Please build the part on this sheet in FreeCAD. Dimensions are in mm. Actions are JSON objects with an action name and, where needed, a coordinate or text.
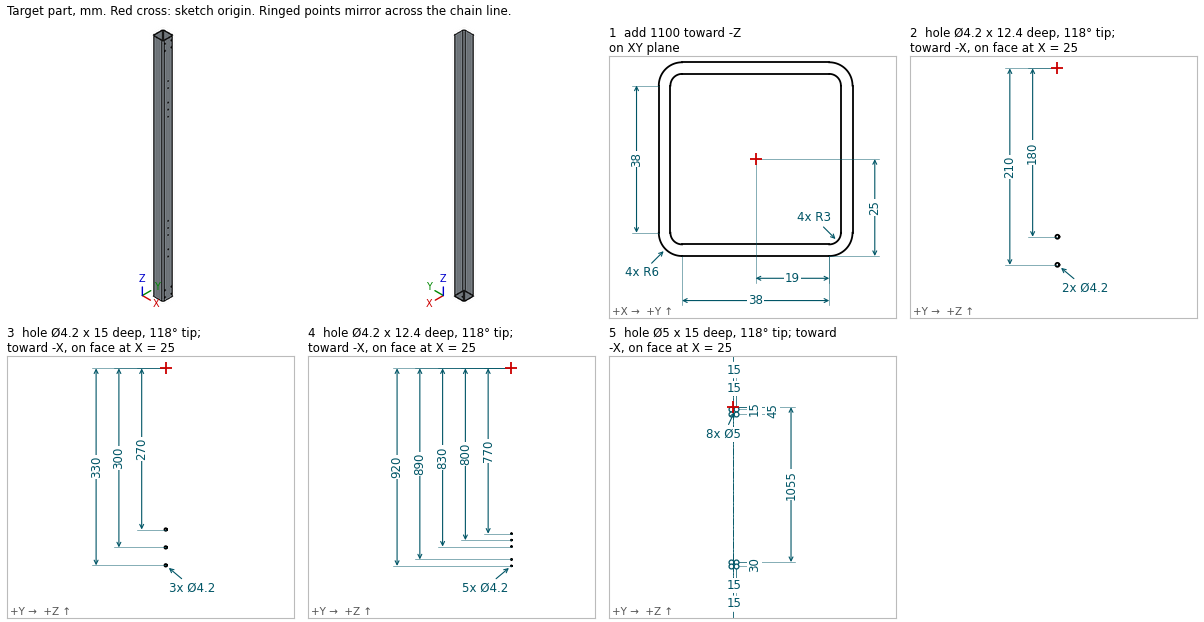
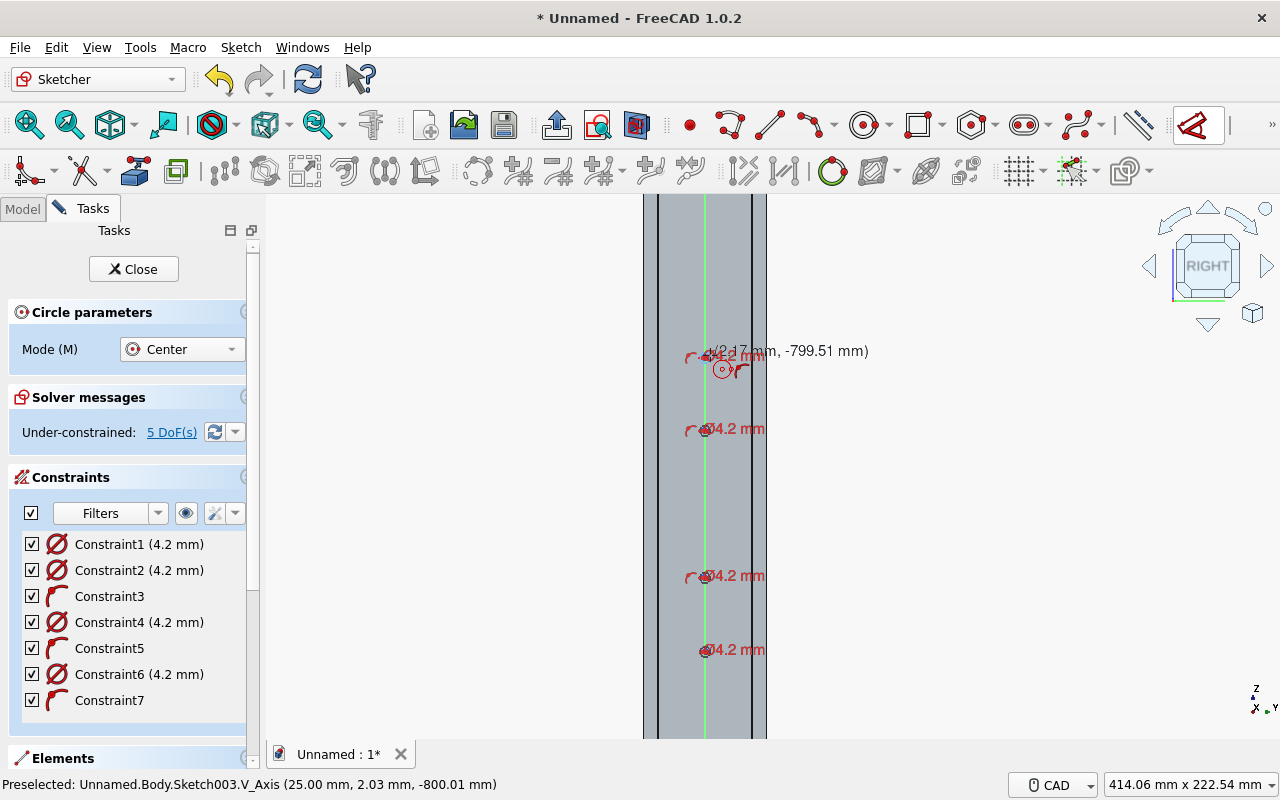
{"action": "scroll", "coordinate": [705, 283], "scroll_direction": "up", "scroll_amount": 8}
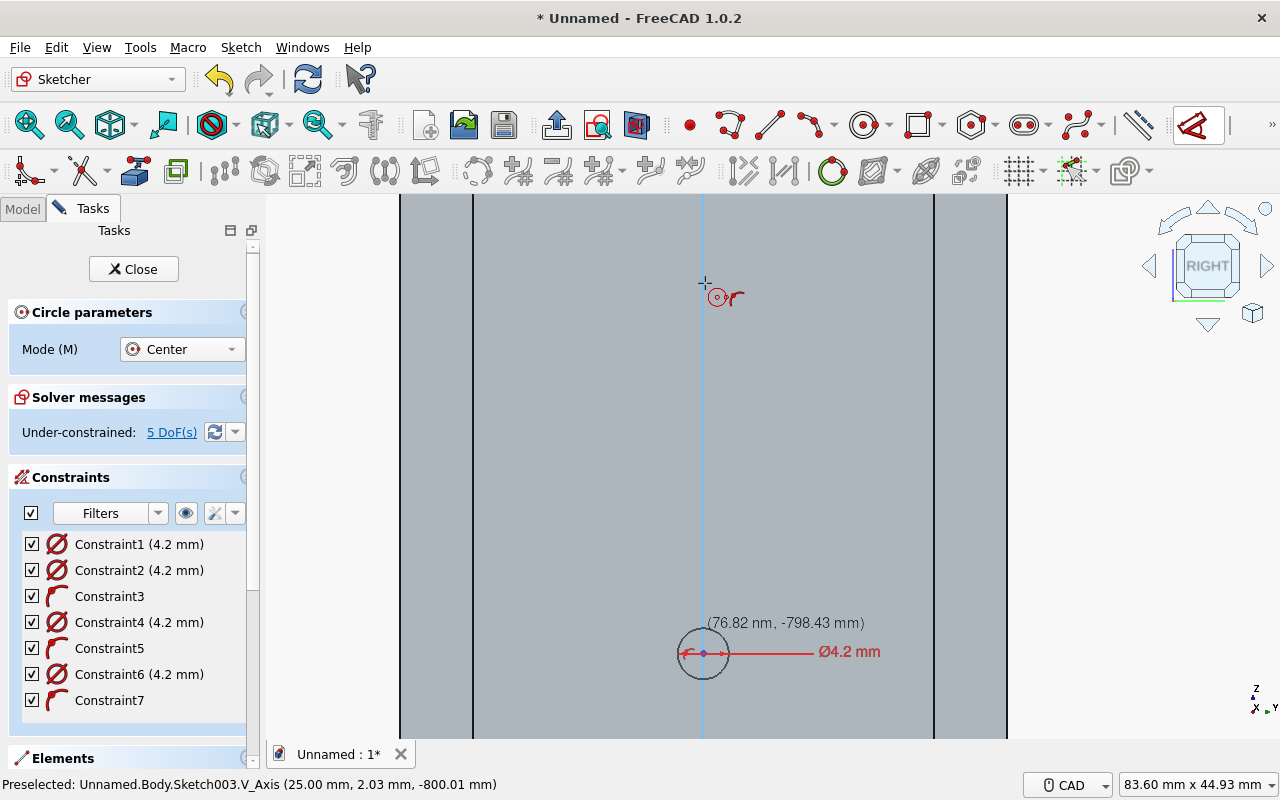
{"action": "scroll", "coordinate": [705, 283], "scroll_direction": "down", "scroll_amount": 8}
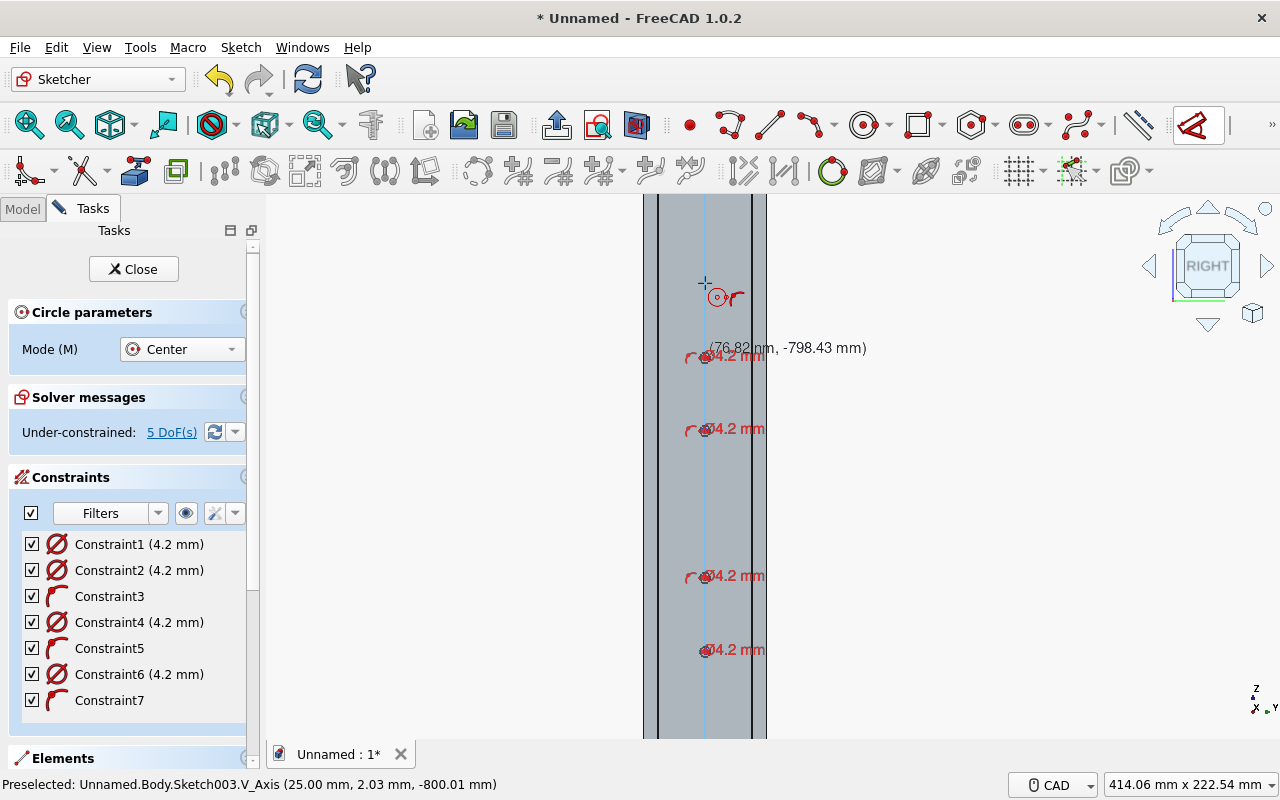
{"action": "left_click", "coordinate": [705, 283]}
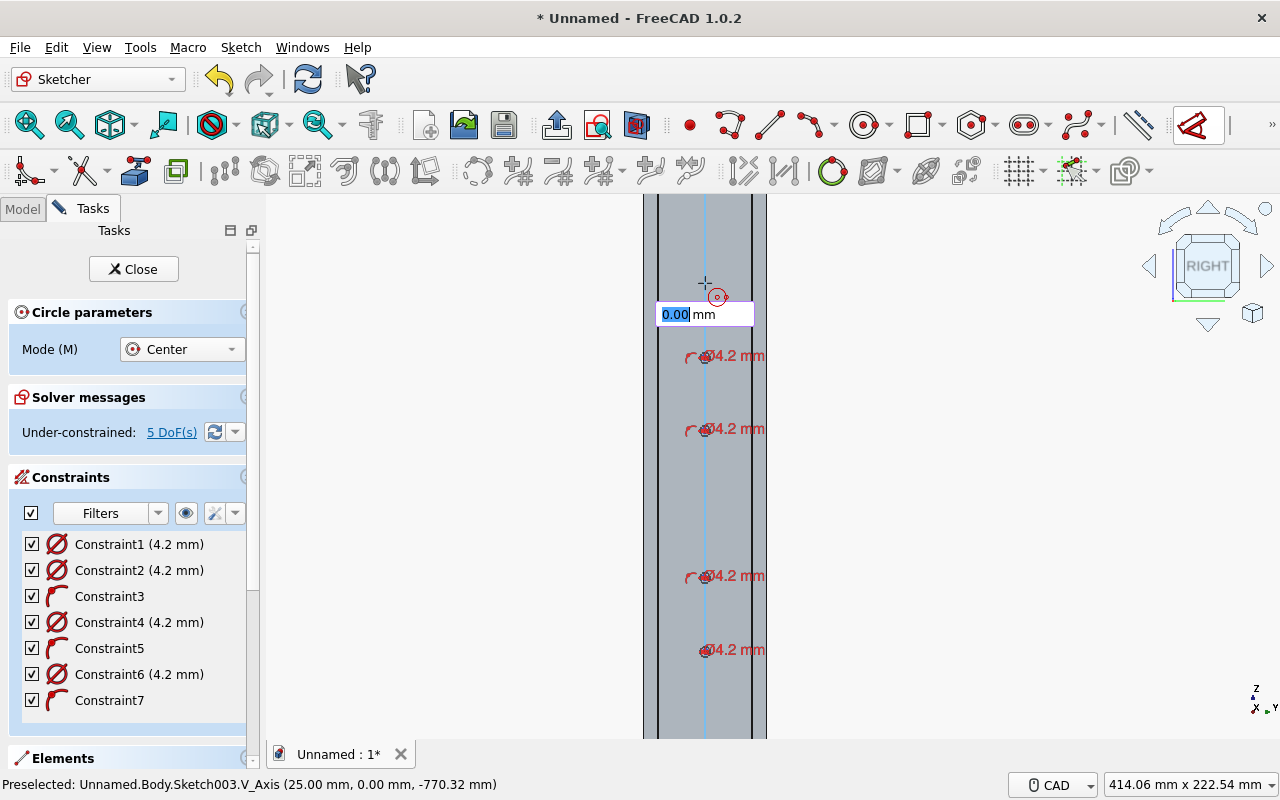
{"action": "scroll", "coordinate": [710, 281], "scroll_direction": "up", "scroll_amount": 6}
{"action": "mouse_move", "coordinate": [708, 282]}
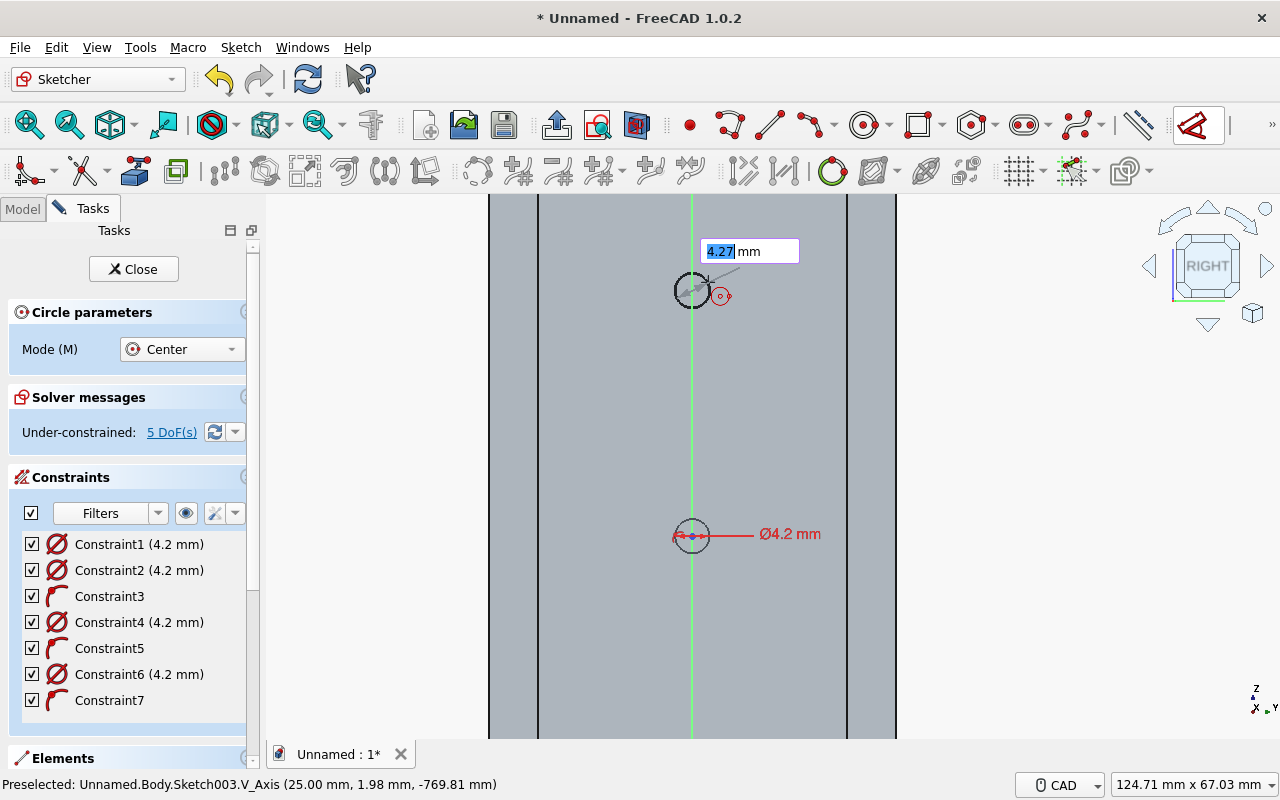
{"action": "type", "text": "4.2"}
{"action": "key", "text": "Return"}
{"action": "key", "text": "Escape"}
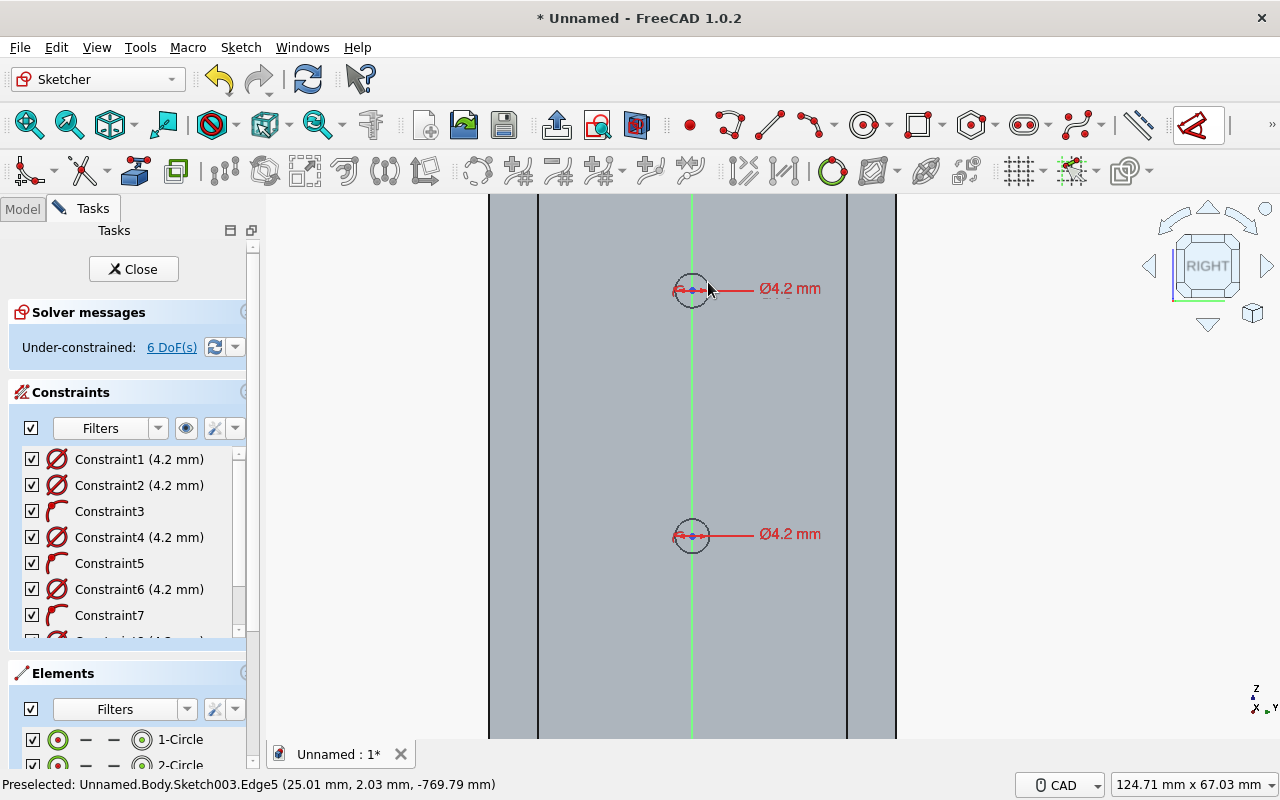
{"action": "scroll", "coordinate": [710, 281], "scroll_direction": "down", "scroll_amount": 6}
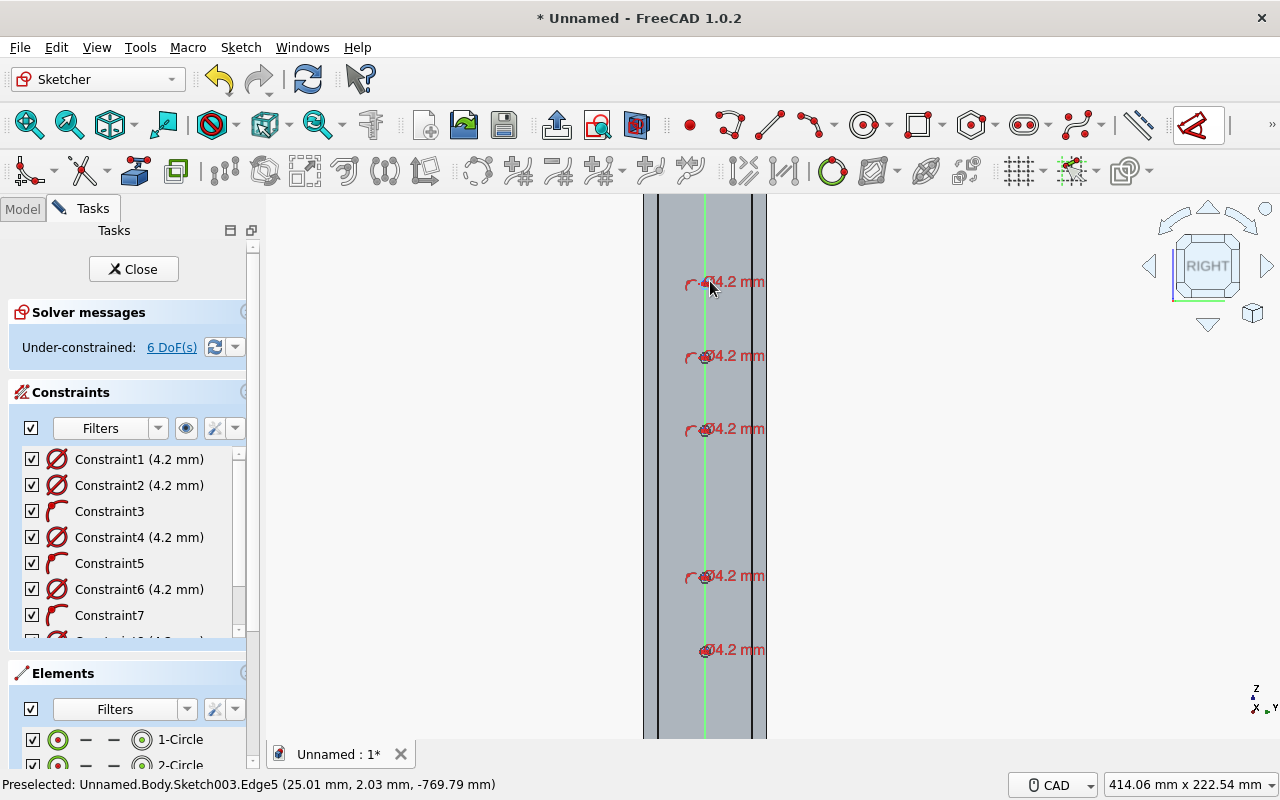
{"action": "left_click", "coordinate": [705, 652]}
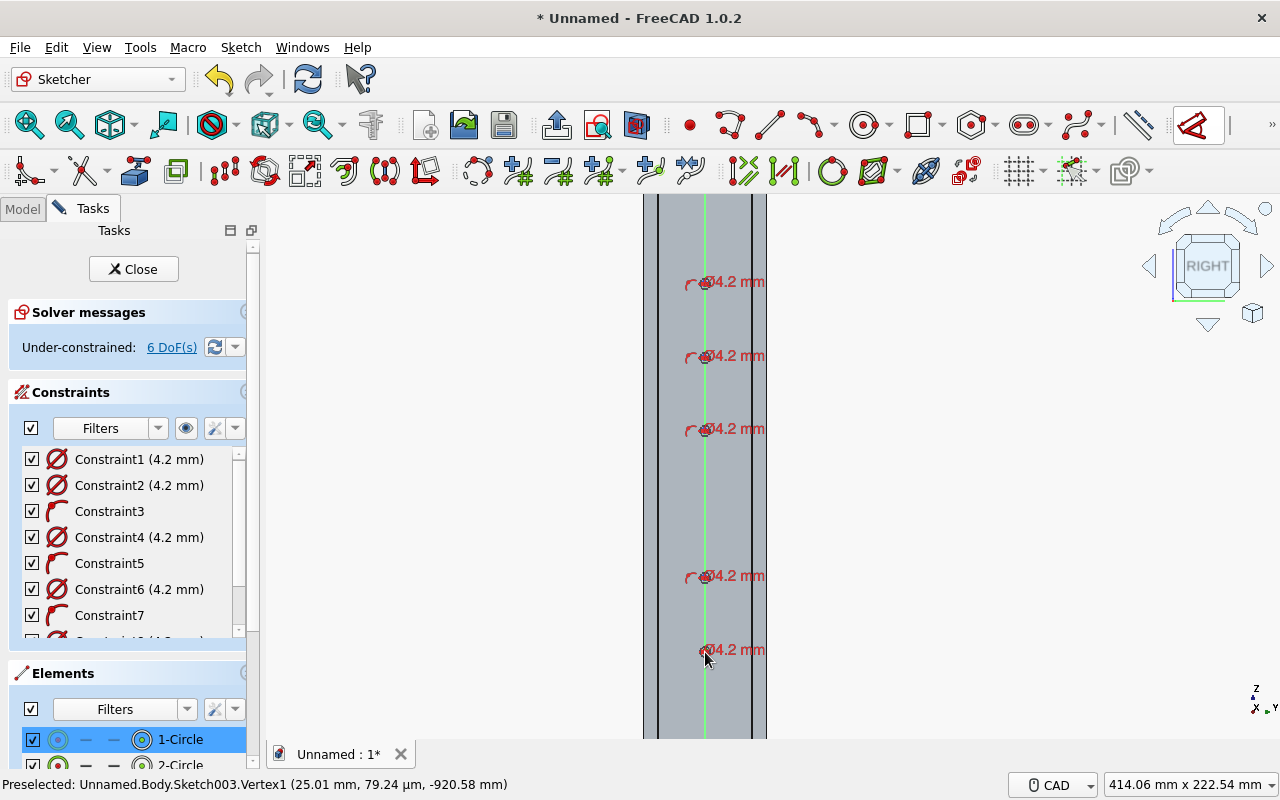
{"action": "left_click", "coordinate": [705, 536]}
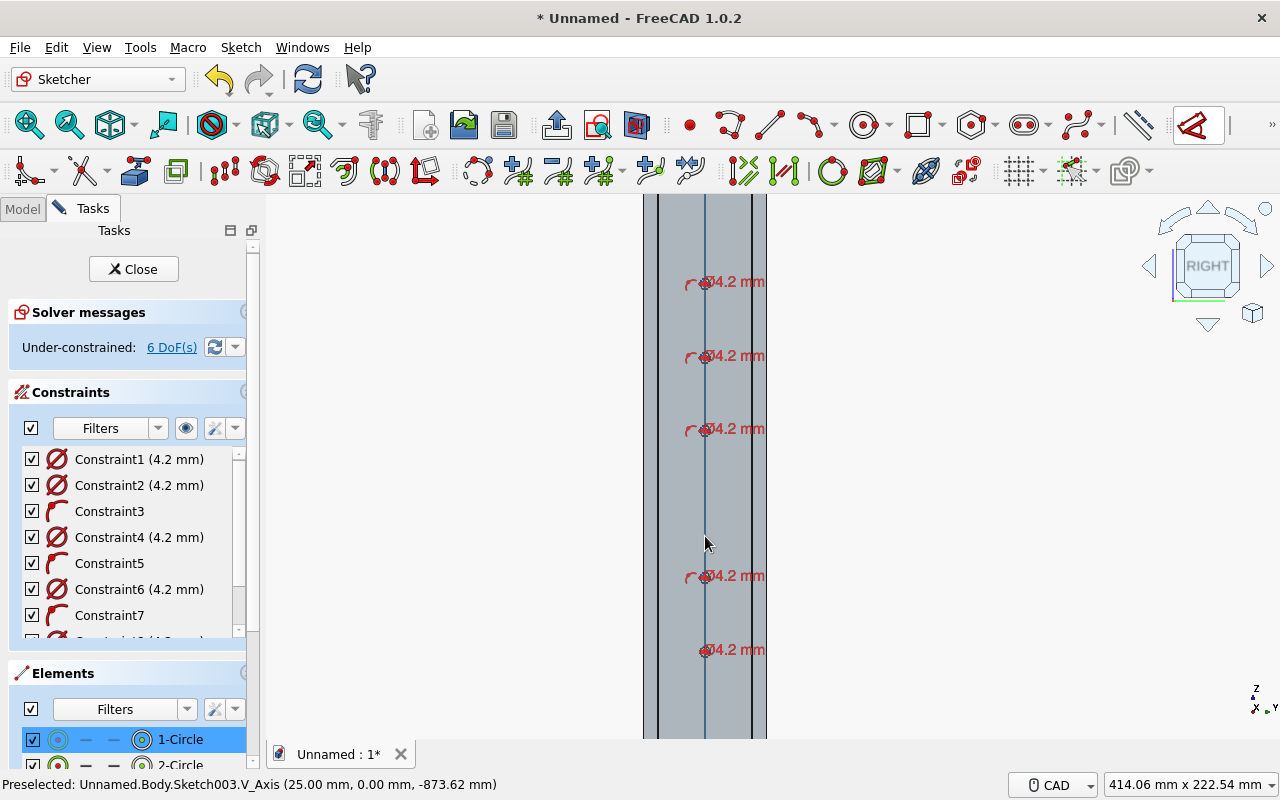
{"action": "key", "text": "c"}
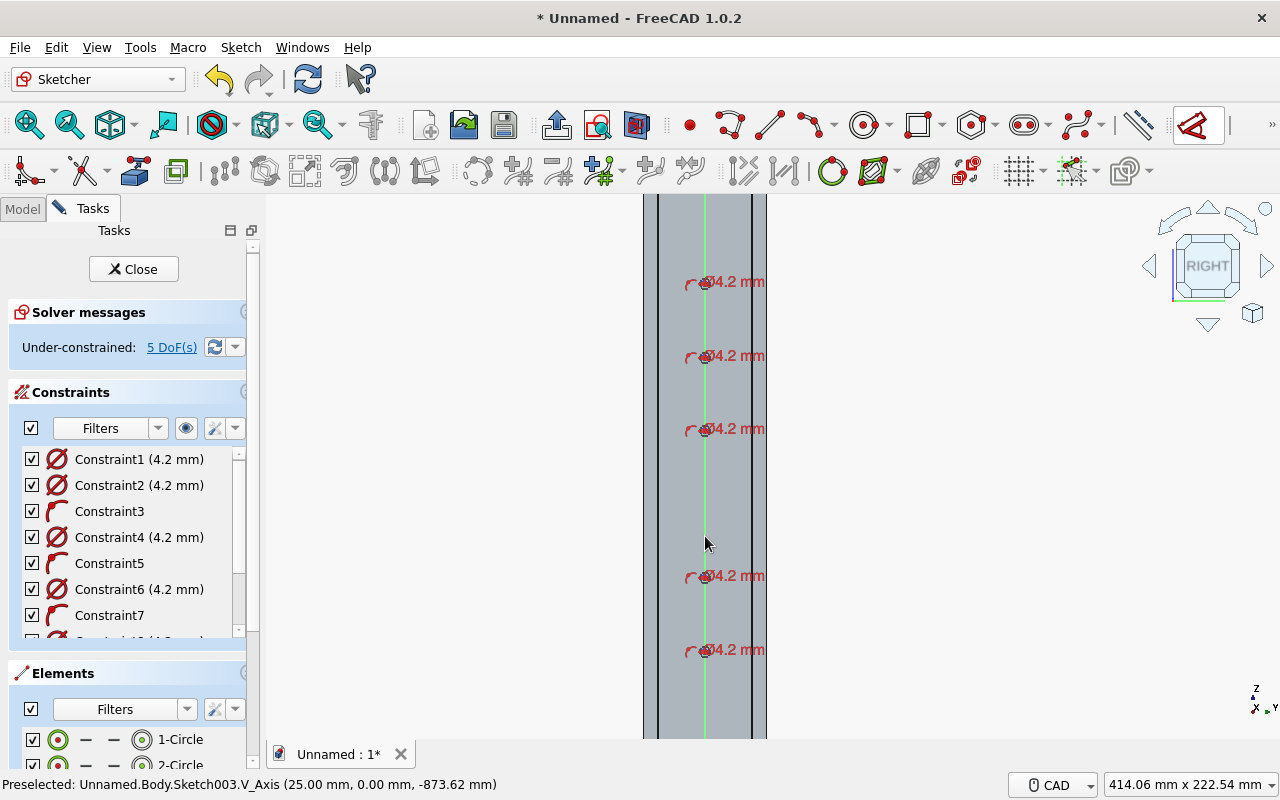
{"action": "left_click", "coordinate": [705, 652]}